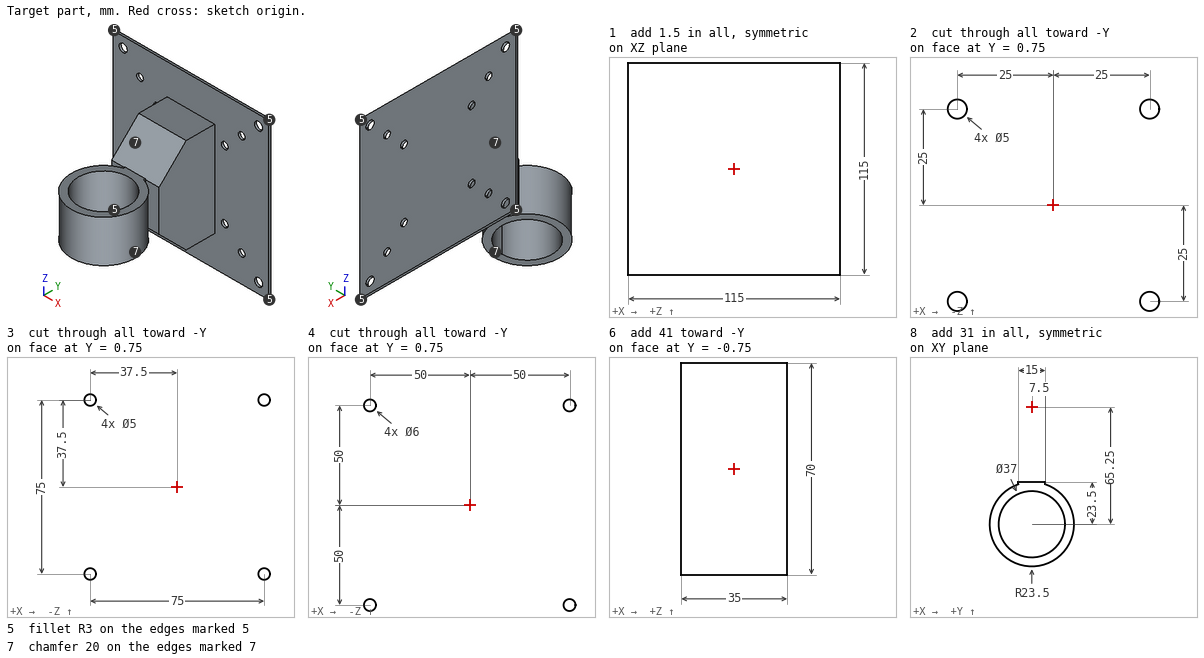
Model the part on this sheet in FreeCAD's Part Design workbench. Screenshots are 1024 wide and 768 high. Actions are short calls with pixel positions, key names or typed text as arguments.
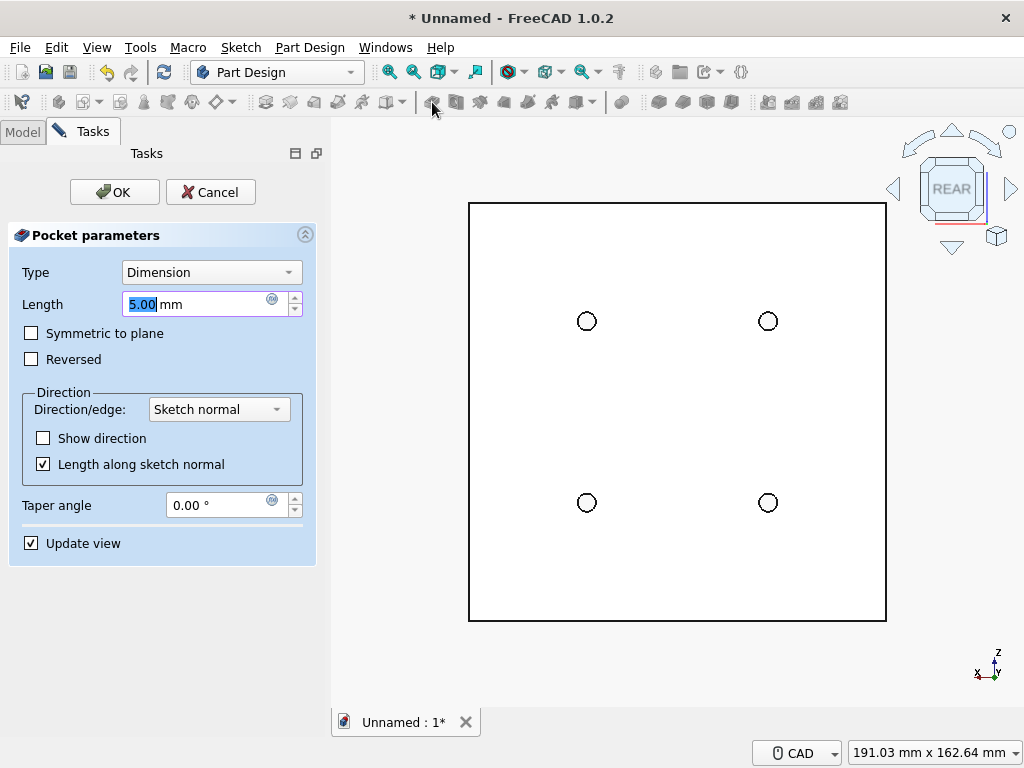
click(212, 272)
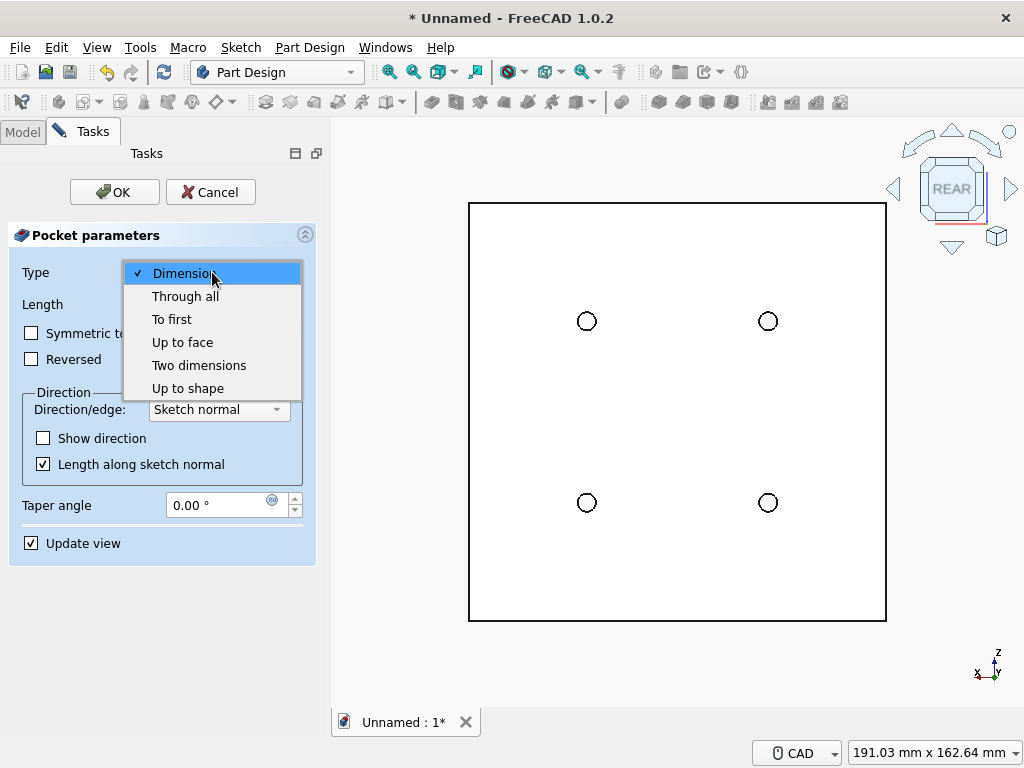
click(212, 296)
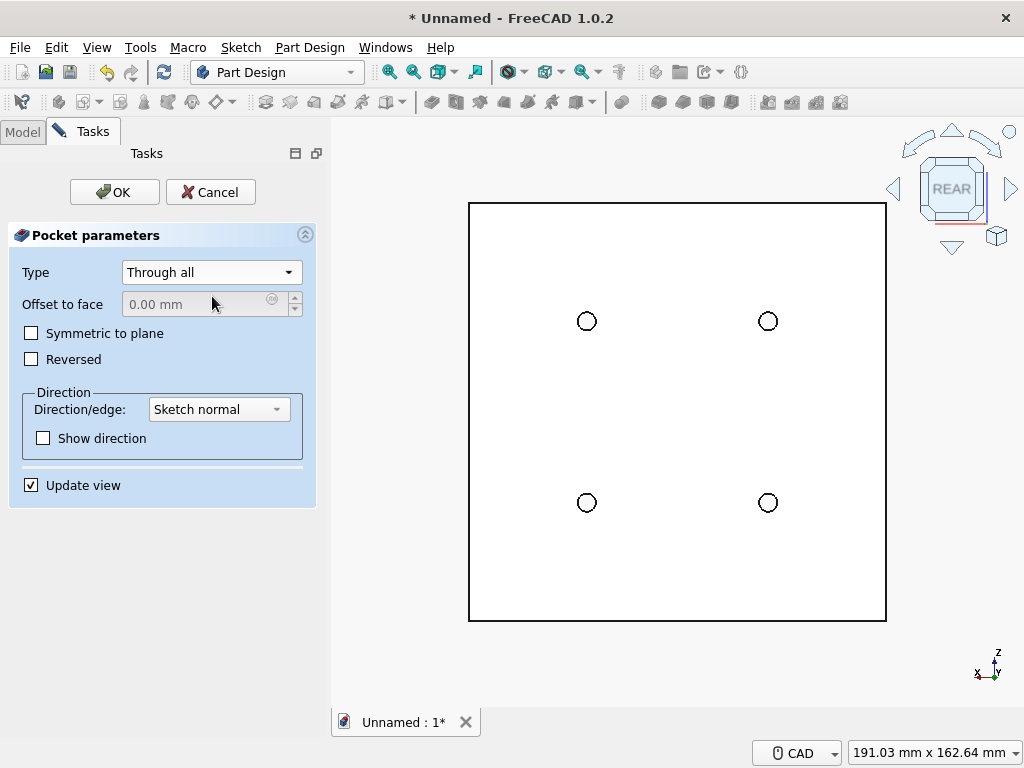
click(115, 192)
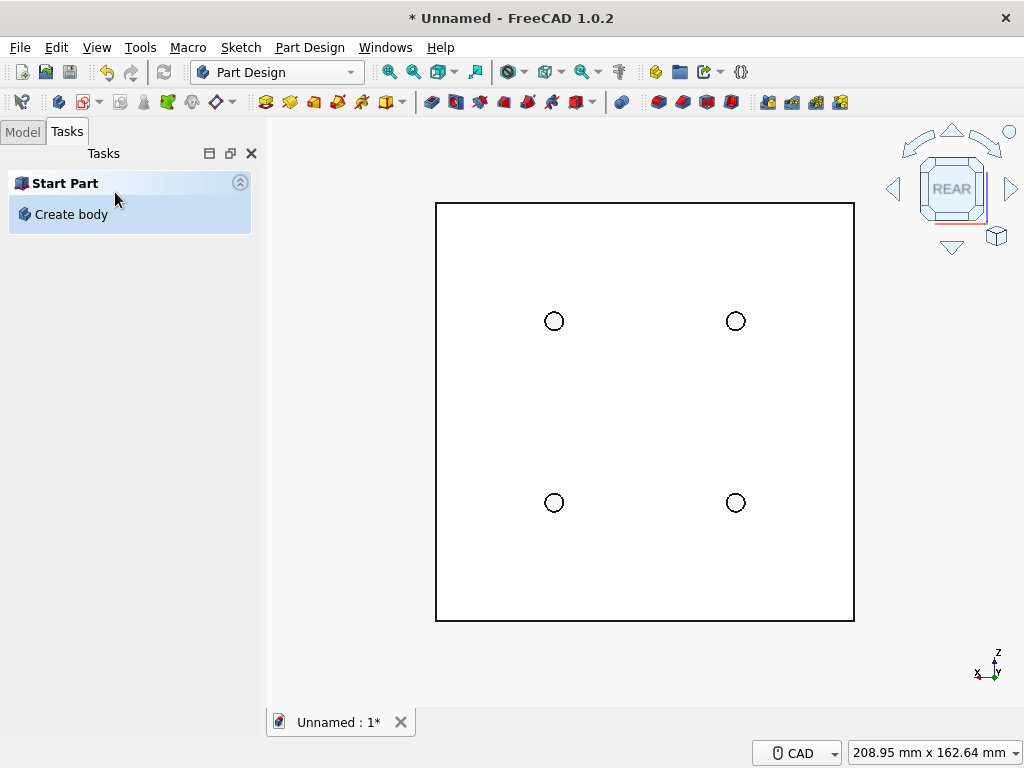
click(645, 411)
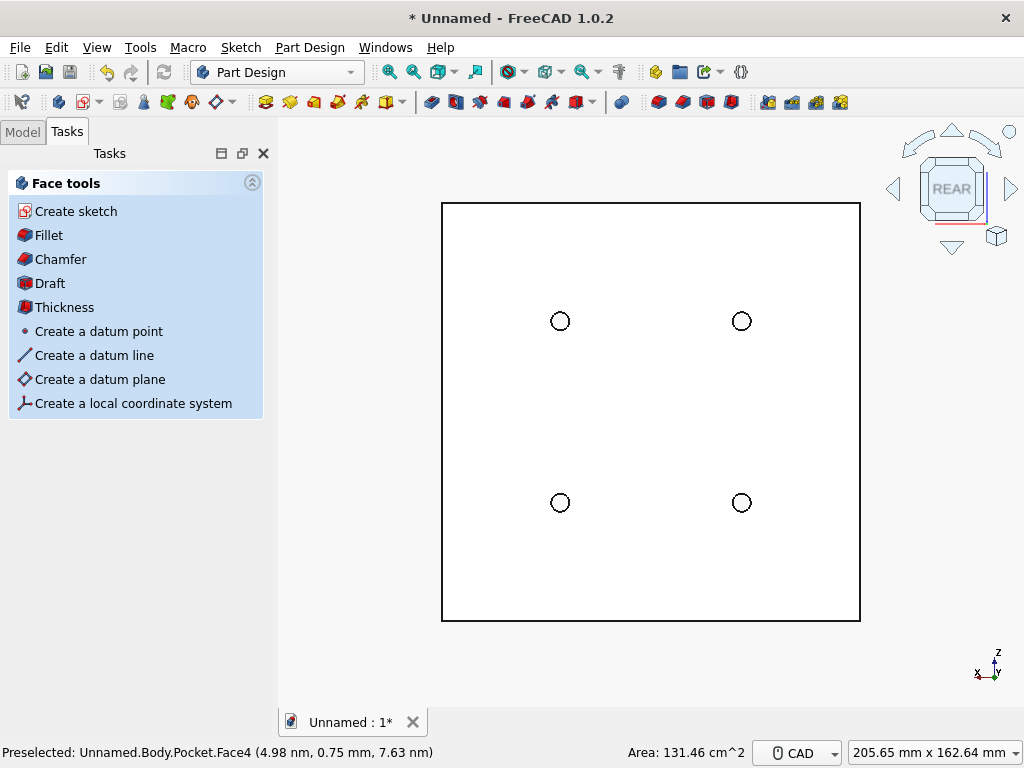
click(84, 102)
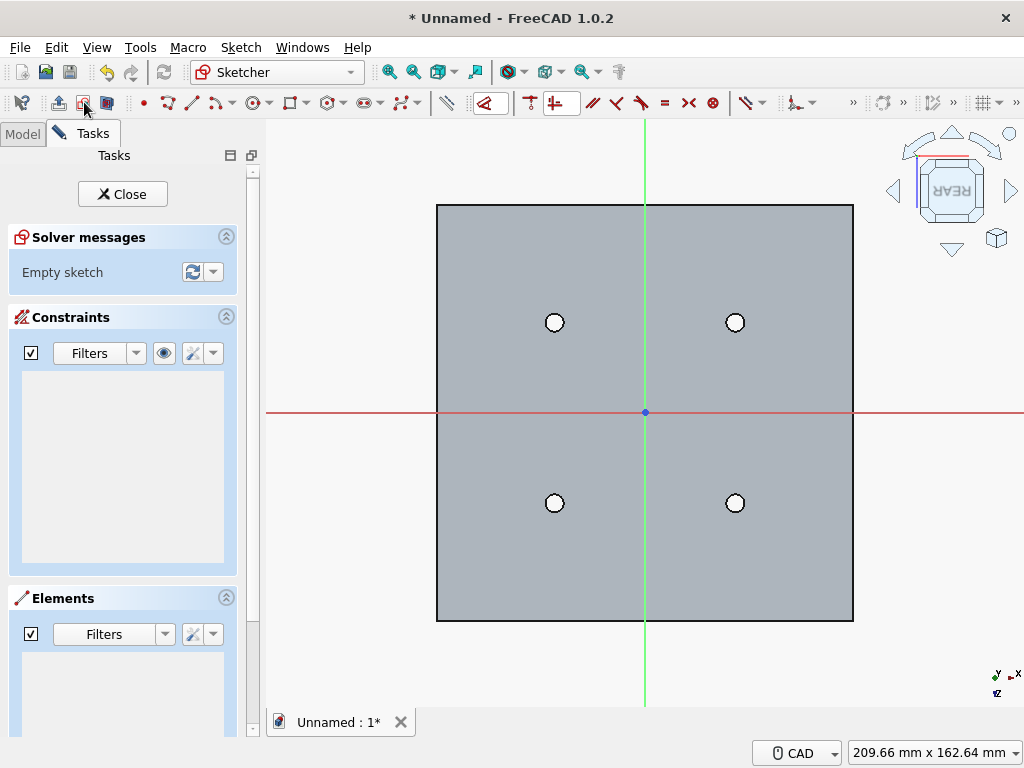
key(g)
key(c)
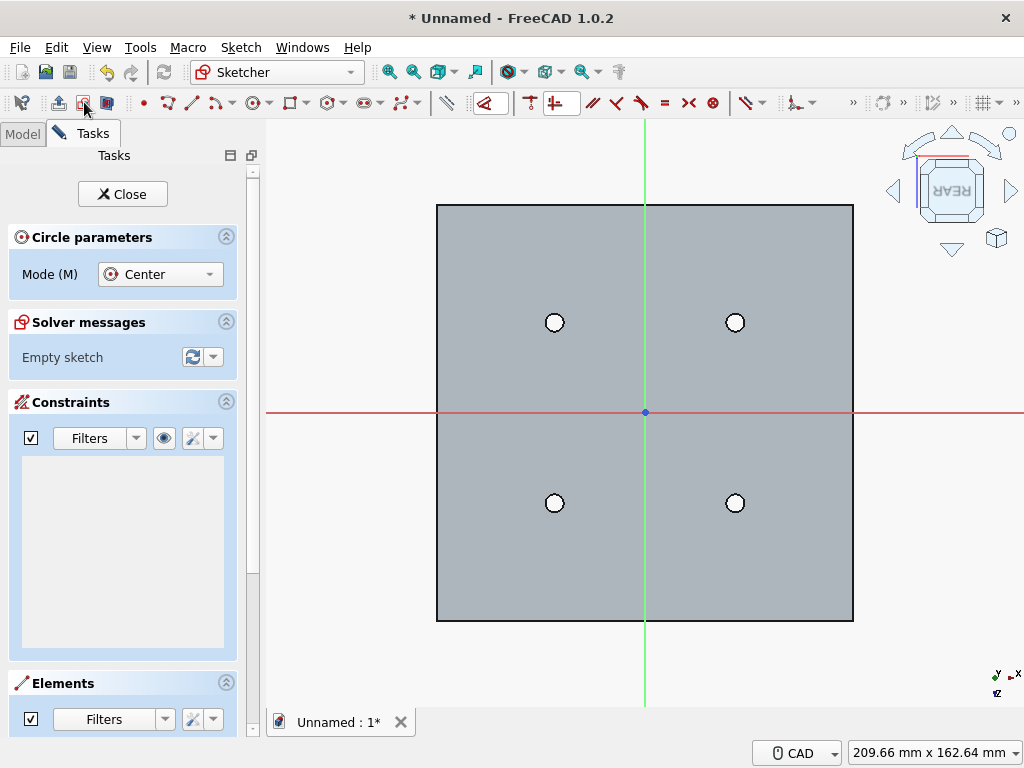
scroll(509, 277, up, 5)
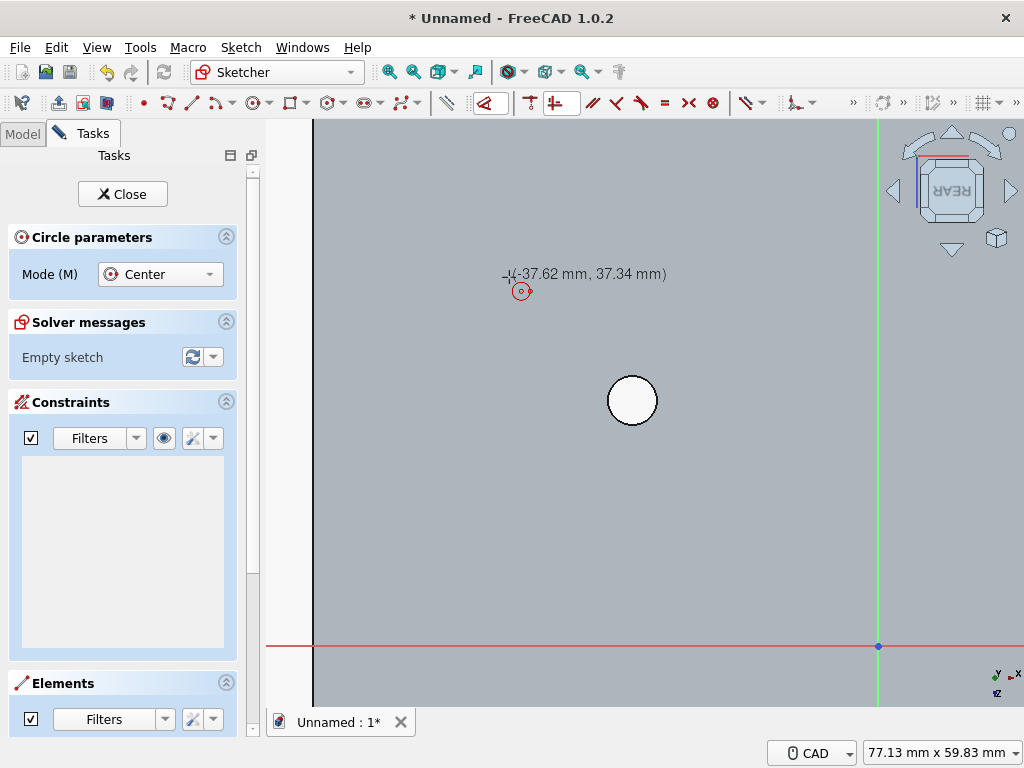
click(510, 278)
click(527, 260)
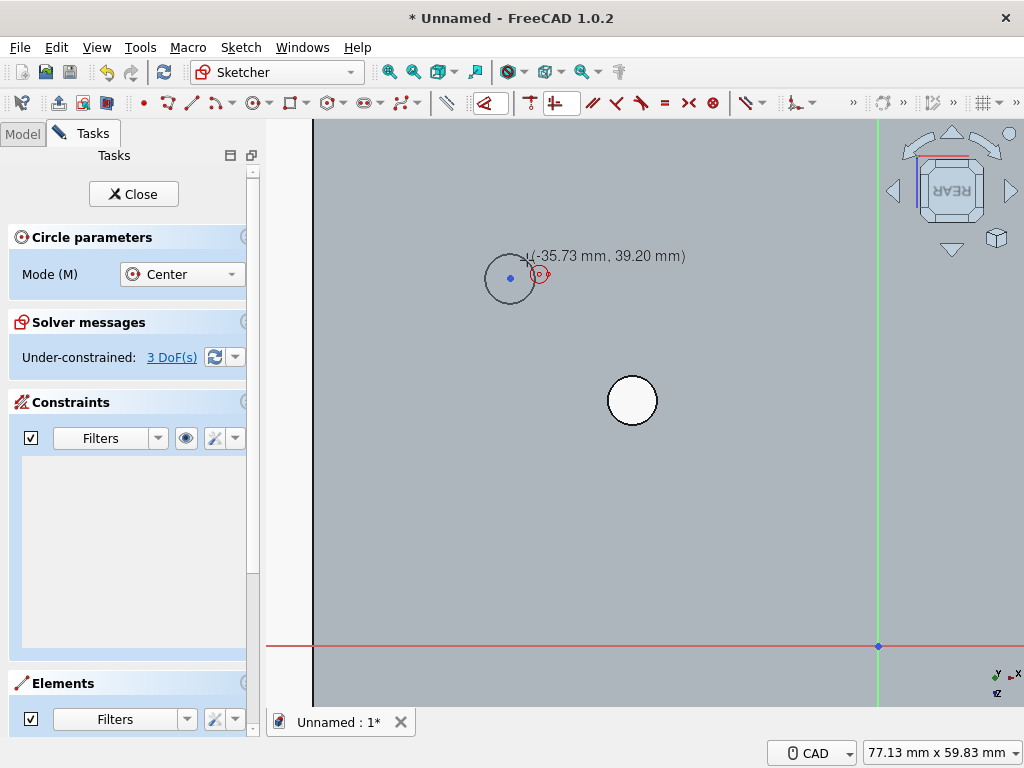
scroll(330, 223, down, 4)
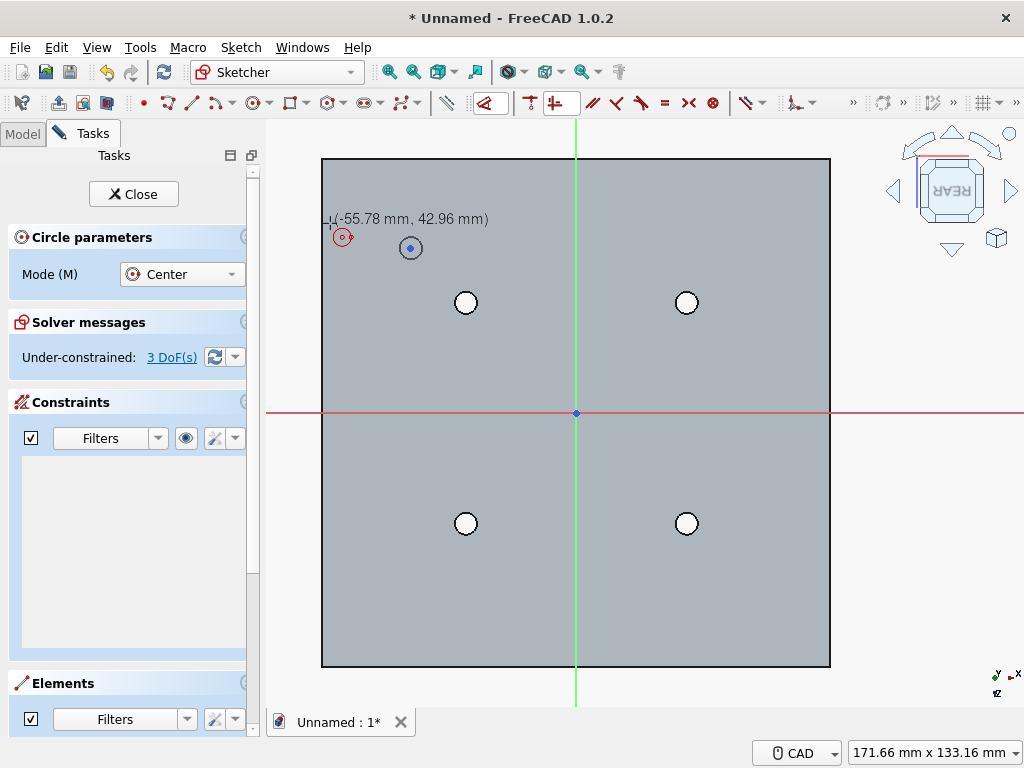
scroll(411, 579, up, 4)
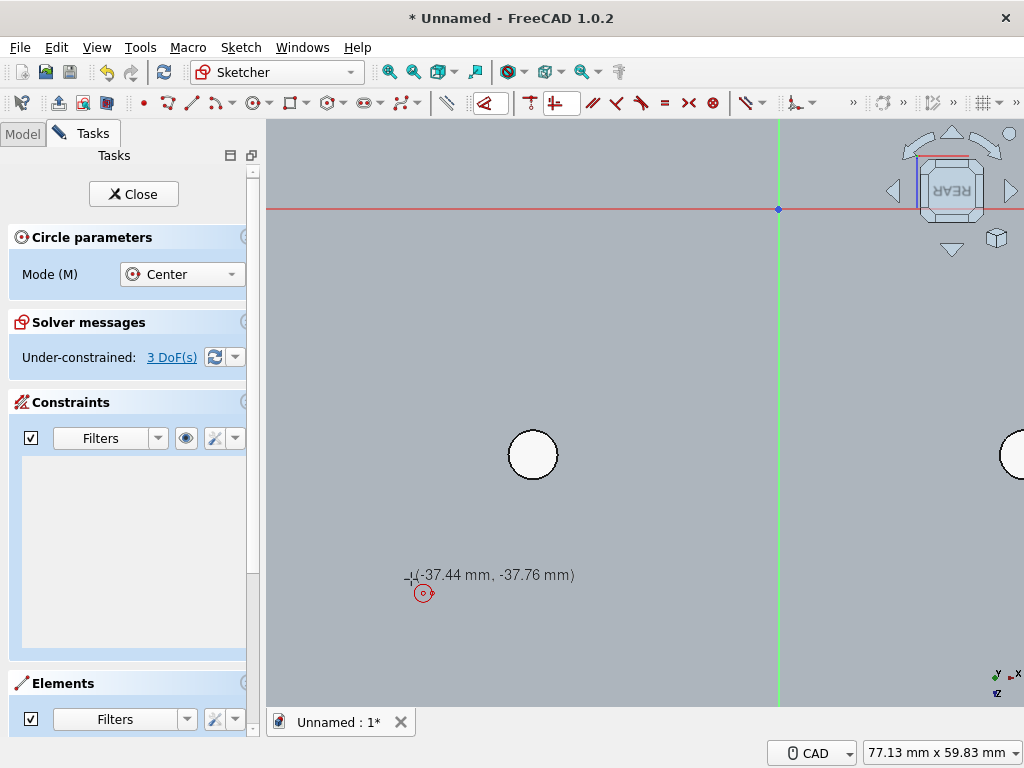
click(410, 578)
click(428, 560)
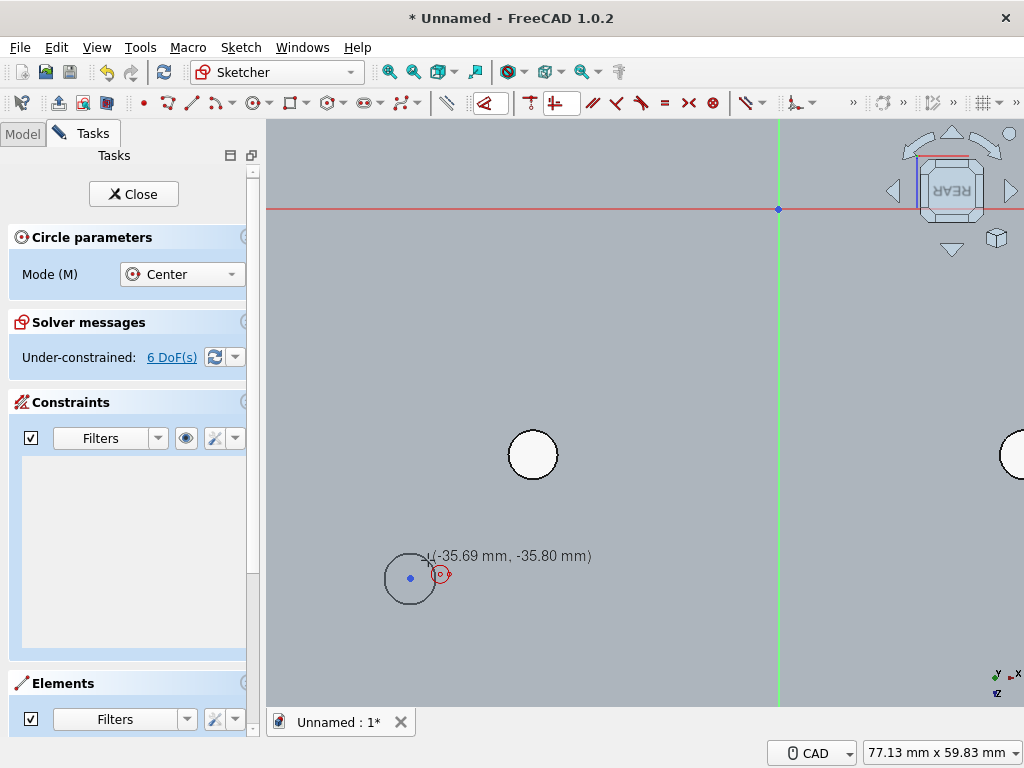
scroll(411, 579, down, 4)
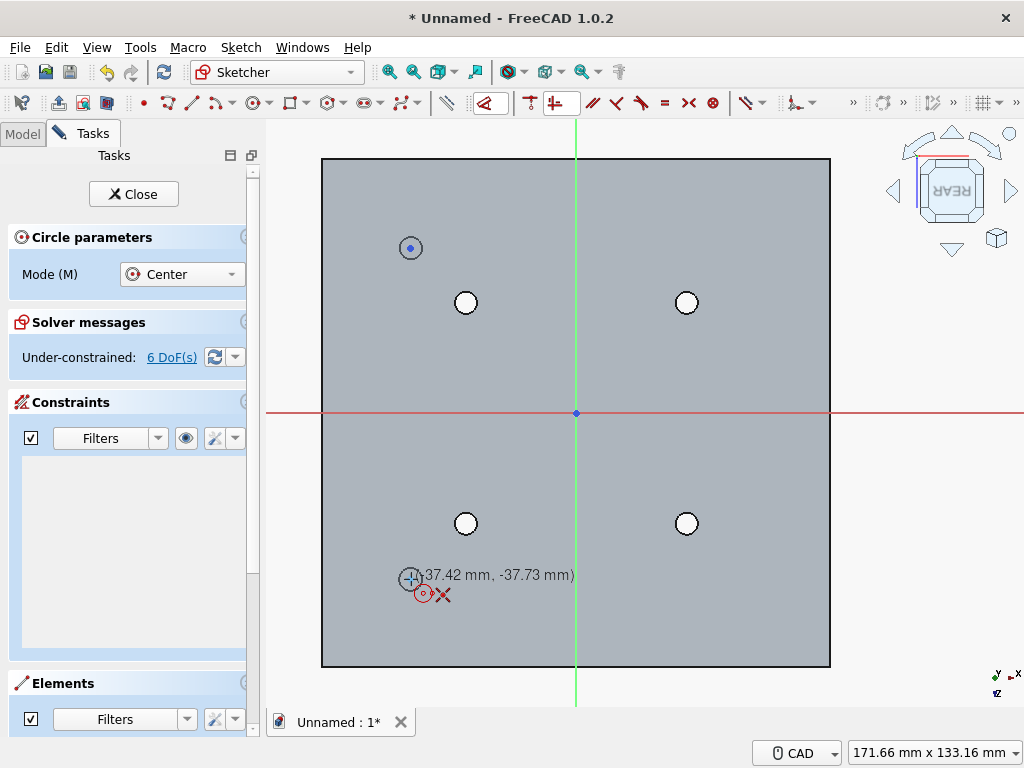
scroll(742, 579, up, 4)